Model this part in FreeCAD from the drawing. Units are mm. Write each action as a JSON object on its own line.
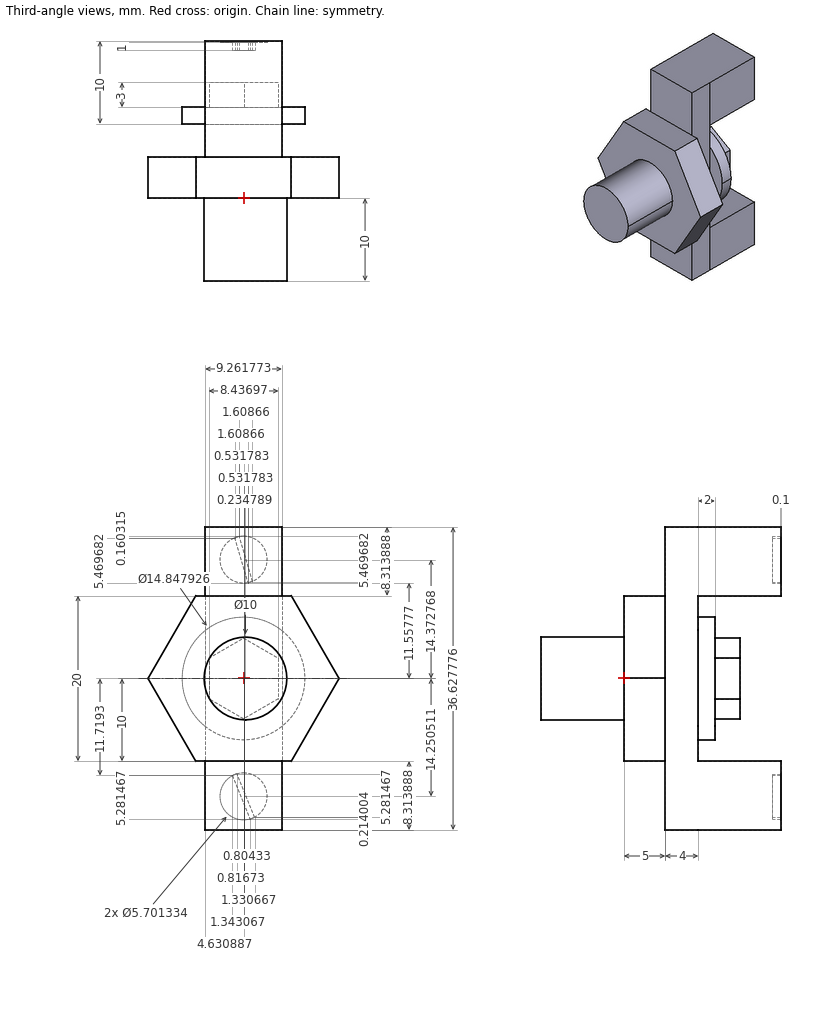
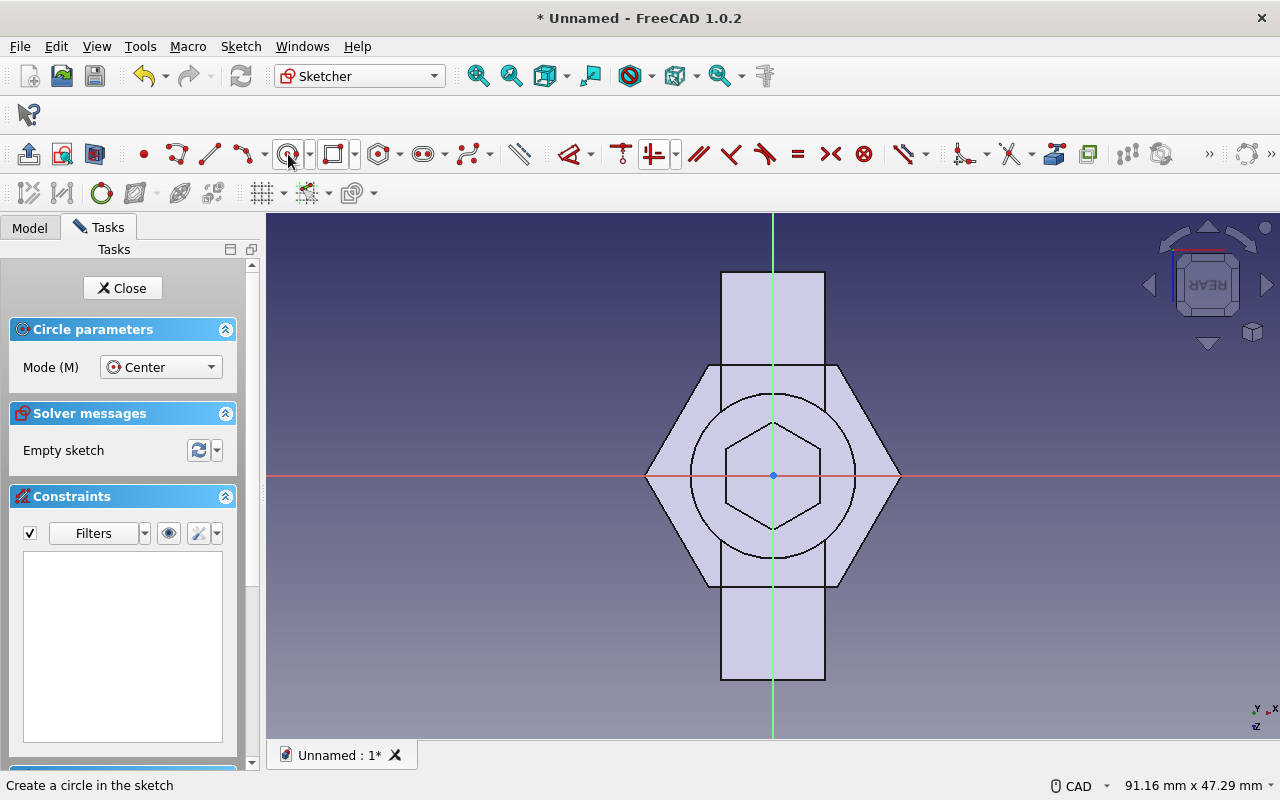
{"action": "left_click", "coordinate": [773, 317]}
{"action": "mouse_move", "coordinate": [795, 295]}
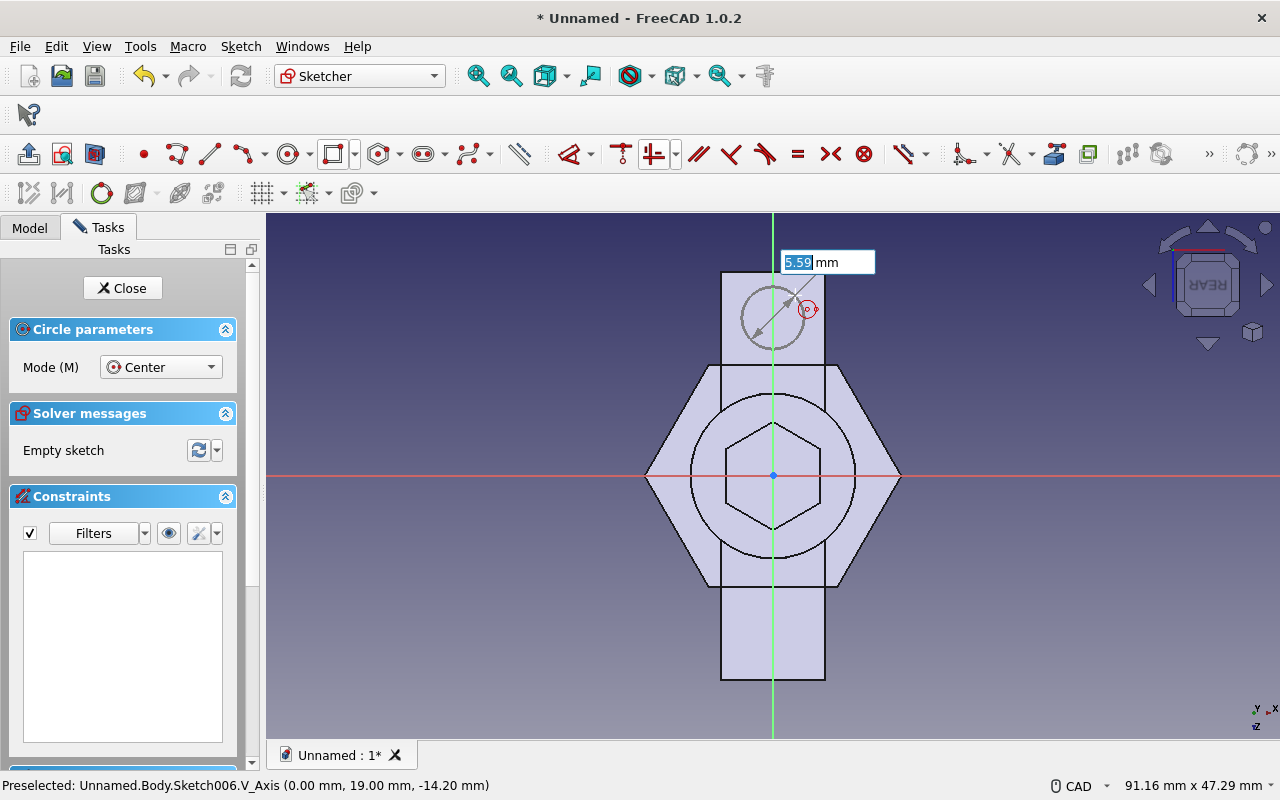
{"action": "type", "text": "5.701334"}
{"action": "key", "text": "Return"}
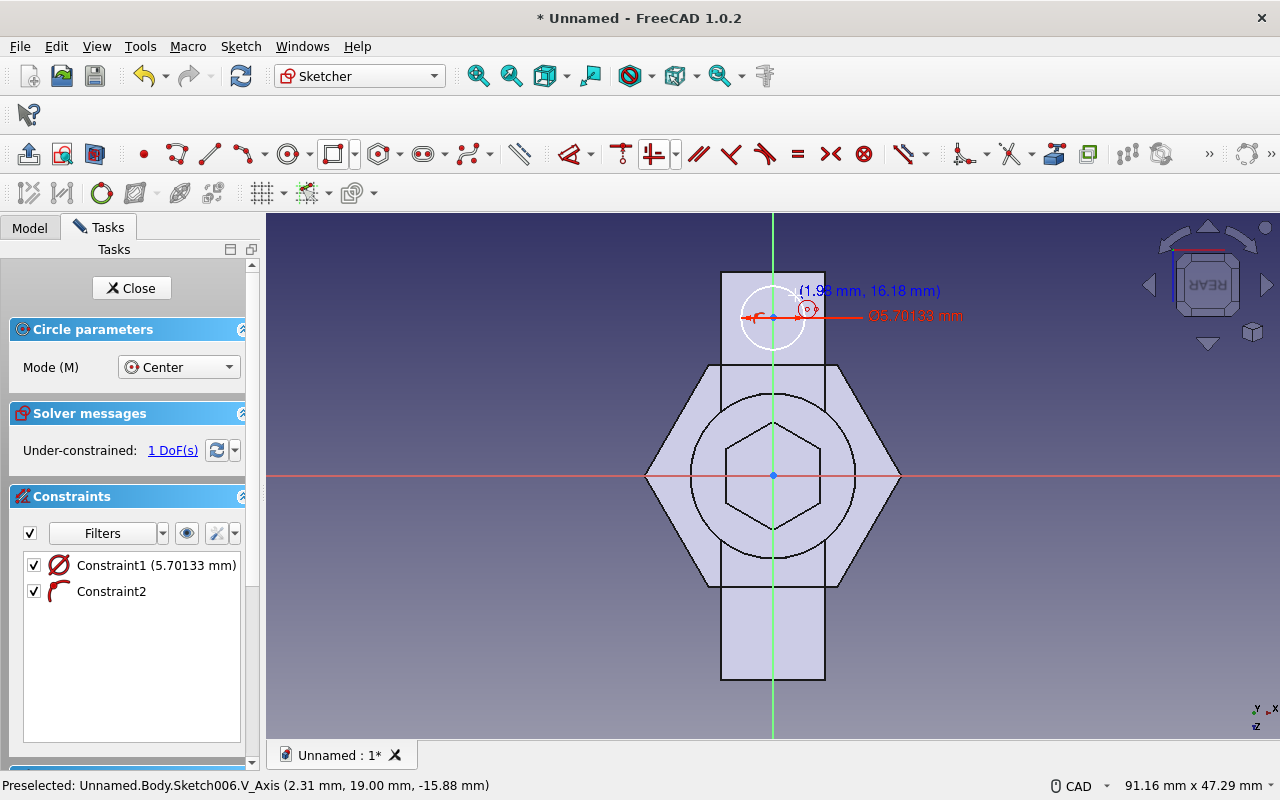
{"action": "left_click", "coordinate": [773, 636]}
{"action": "mouse_move", "coordinate": [795, 613]}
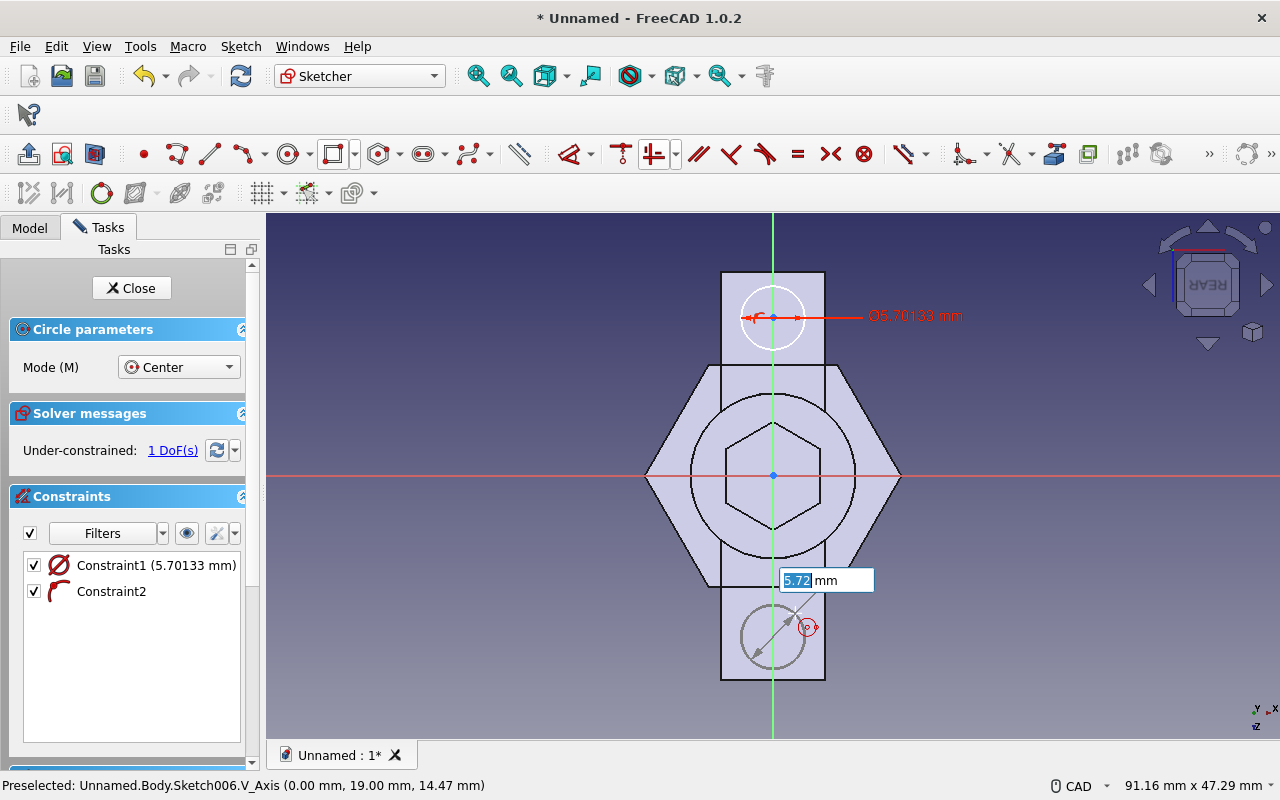
{"action": "type", "text": "5.701334"}
{"action": "key", "text": "Return"}
{"action": "key", "text": "Escape"}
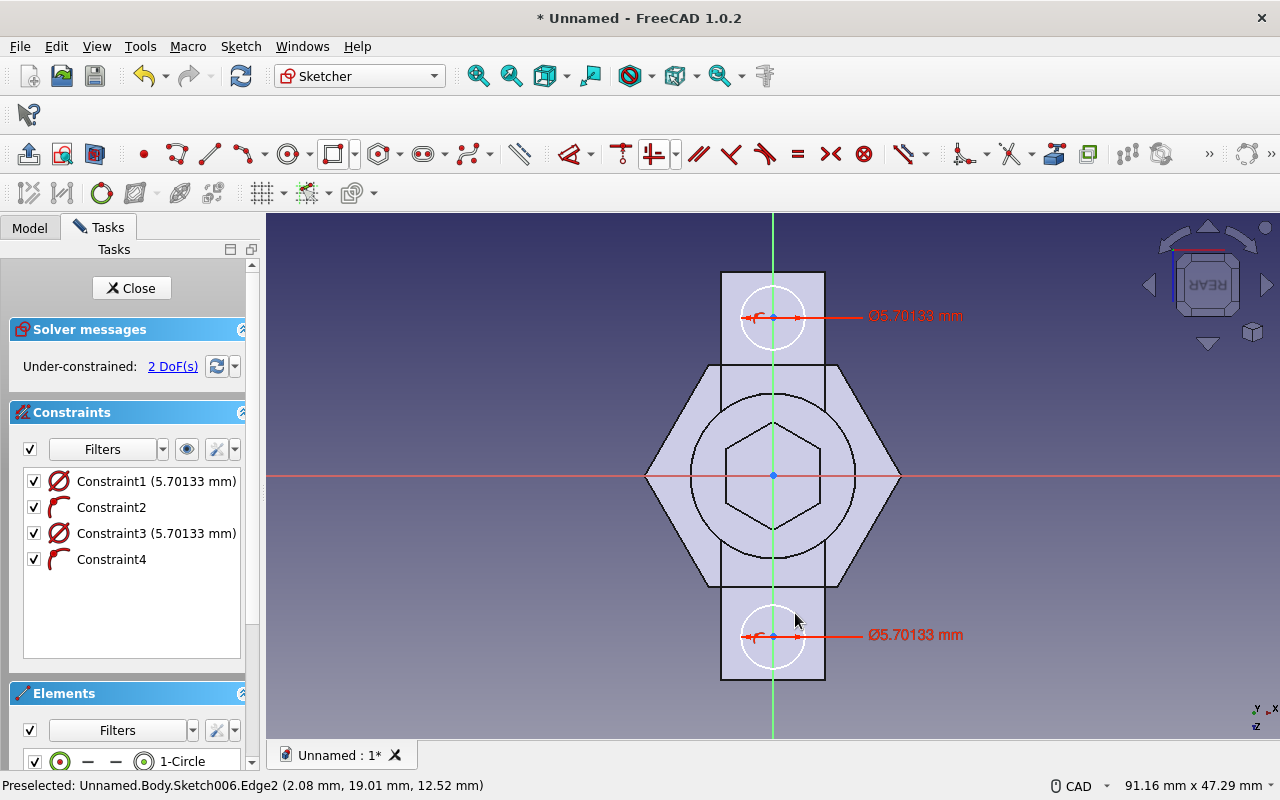
{"action": "left_click", "coordinate": [568, 154]}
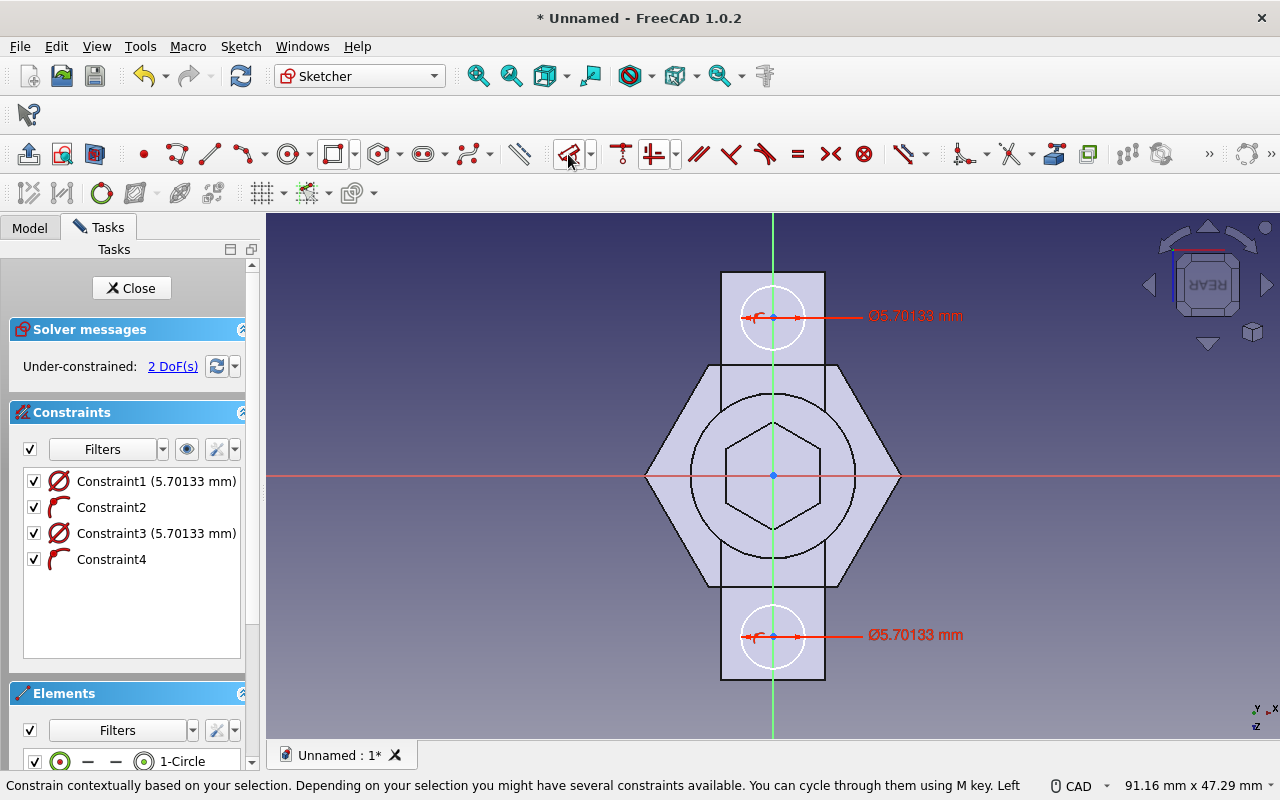
{"action": "left_click", "coordinate": [773, 318]}
{"action": "left_click", "coordinate": [807, 397]}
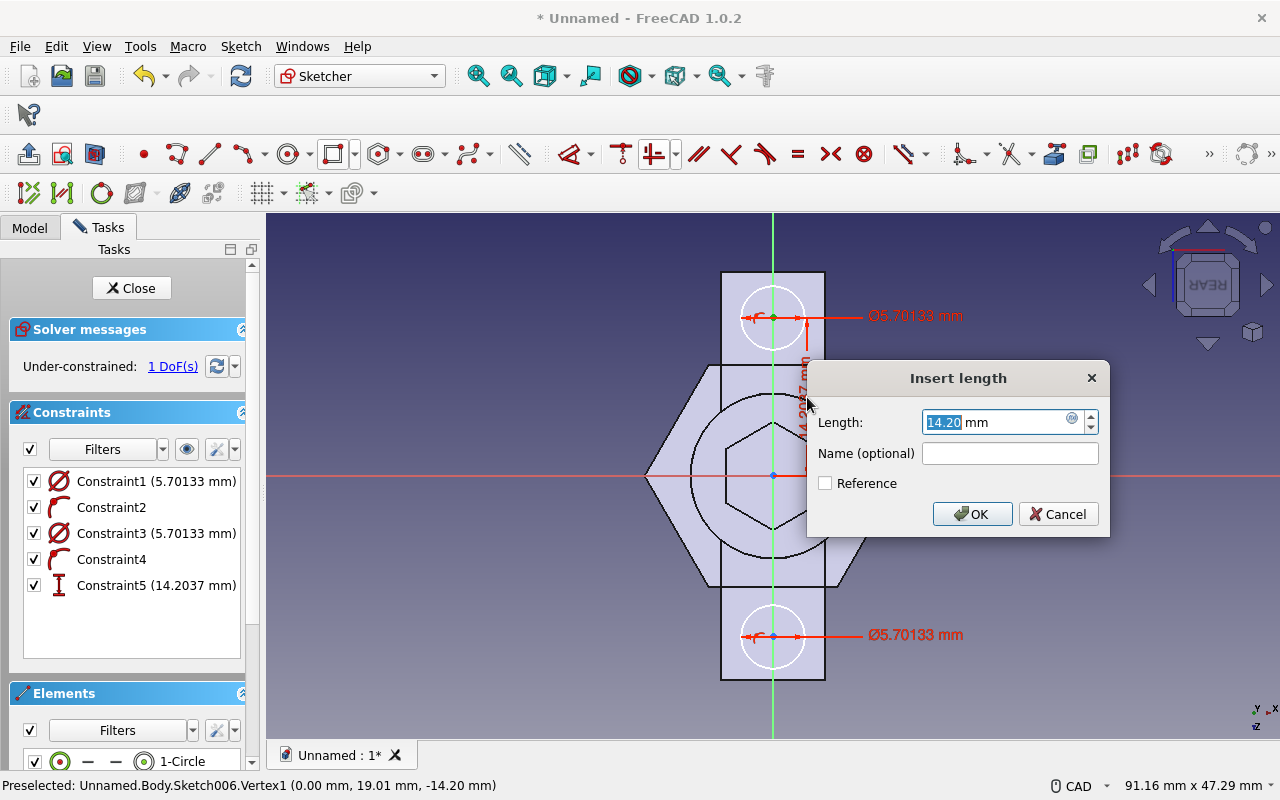
{"action": "type", "text": "14.250511"}
{"action": "key", "text": "Return"}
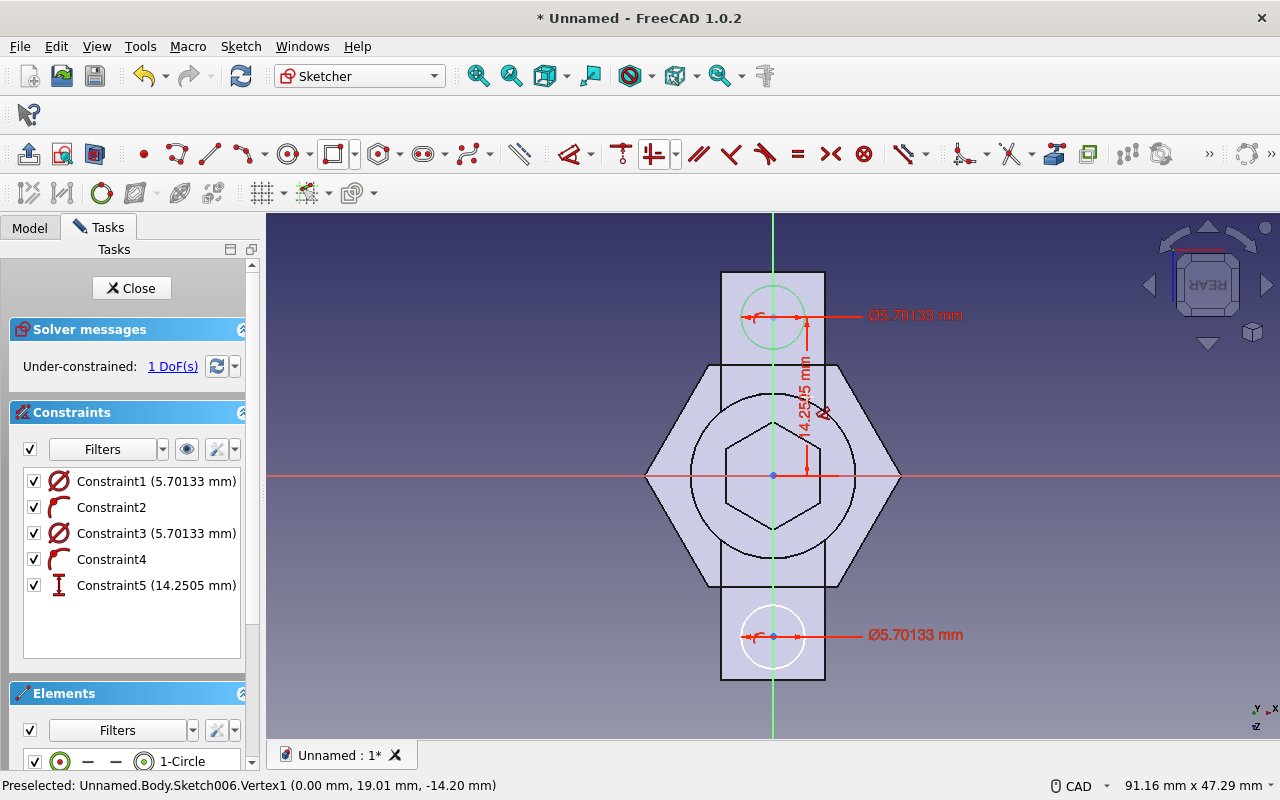
{"action": "left_click", "coordinate": [773, 637]}
{"action": "left_click", "coordinate": [807, 557]}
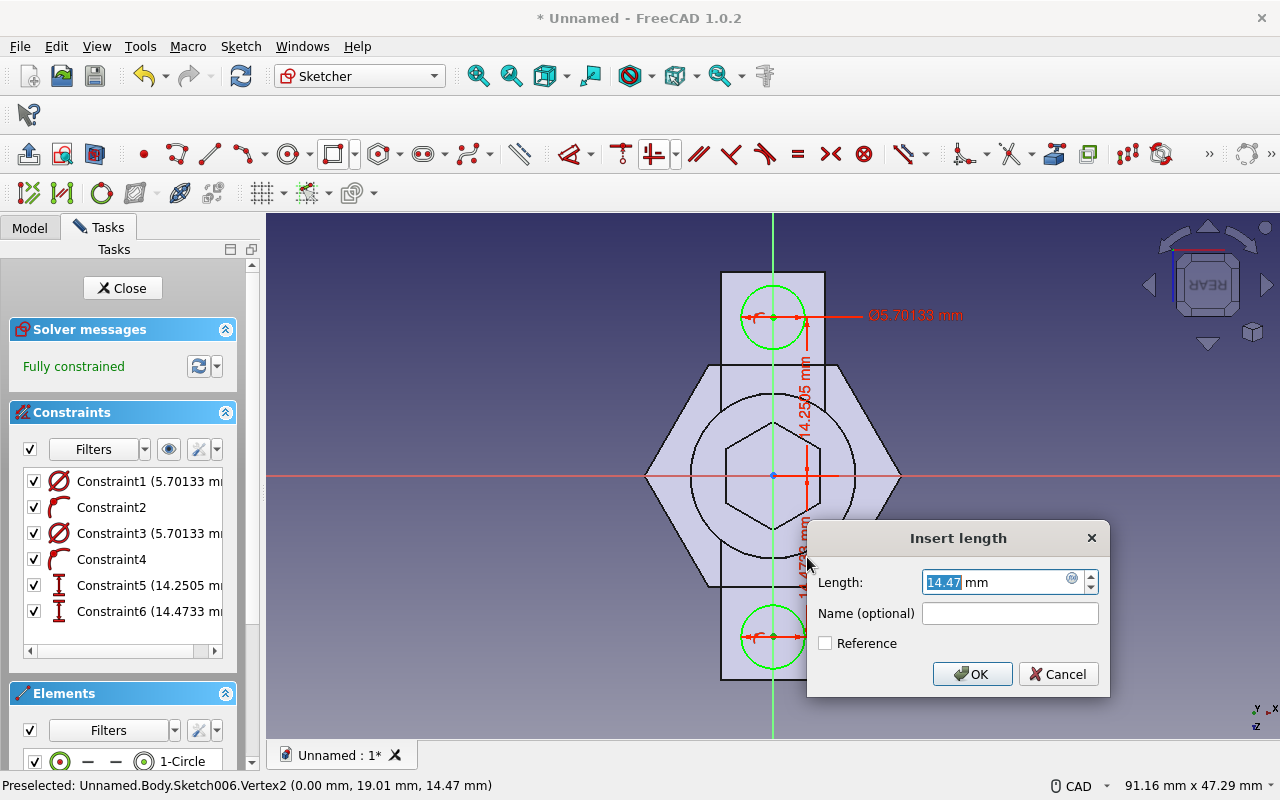
{"action": "type", "text": "14.372768"}
{"action": "key", "text": "Return"}
{"action": "key", "text": "Escape"}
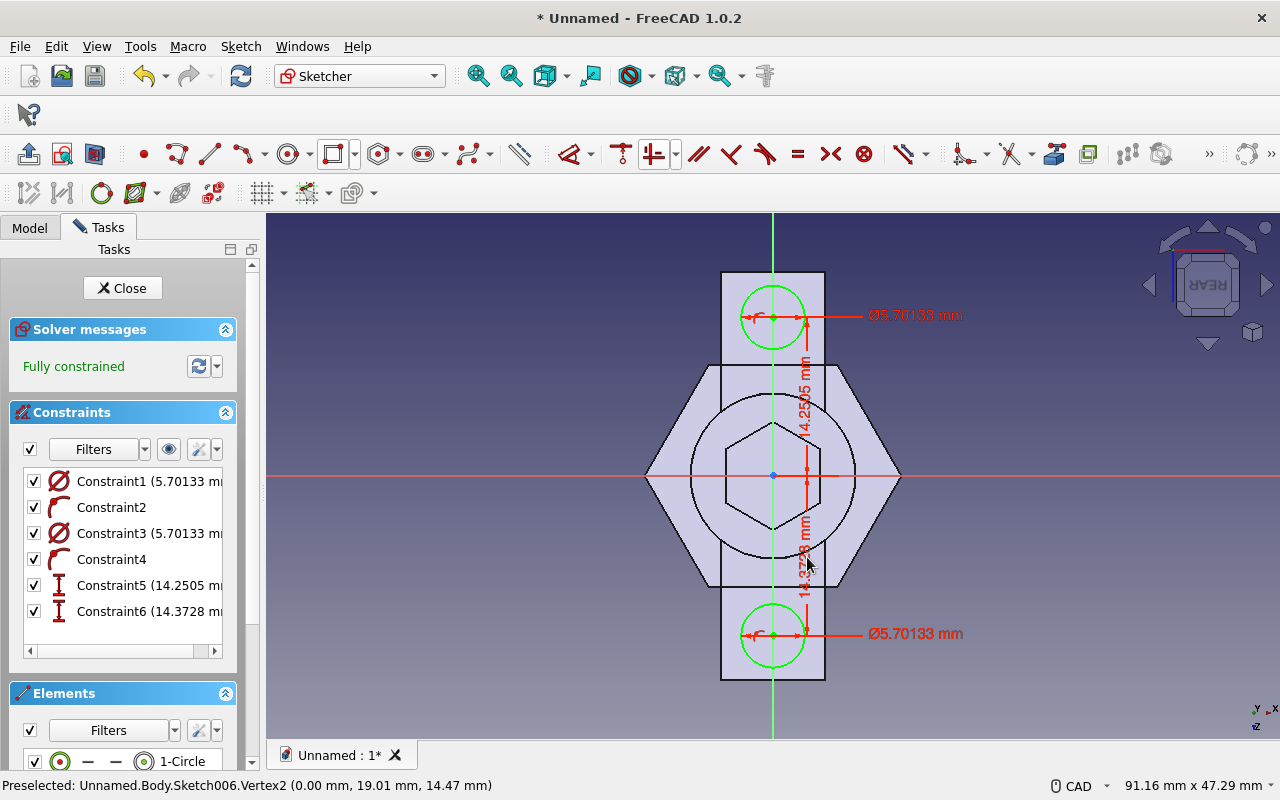
{"action": "left_click", "coordinate": [123, 288]}